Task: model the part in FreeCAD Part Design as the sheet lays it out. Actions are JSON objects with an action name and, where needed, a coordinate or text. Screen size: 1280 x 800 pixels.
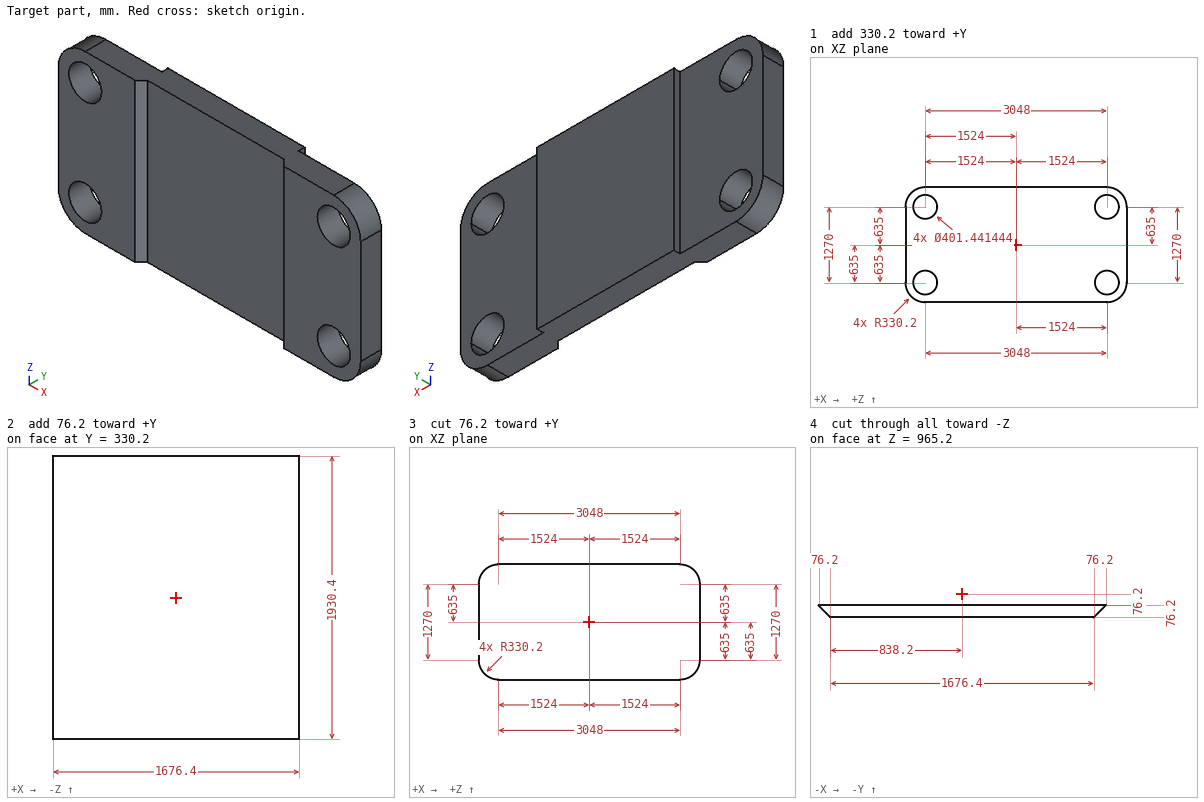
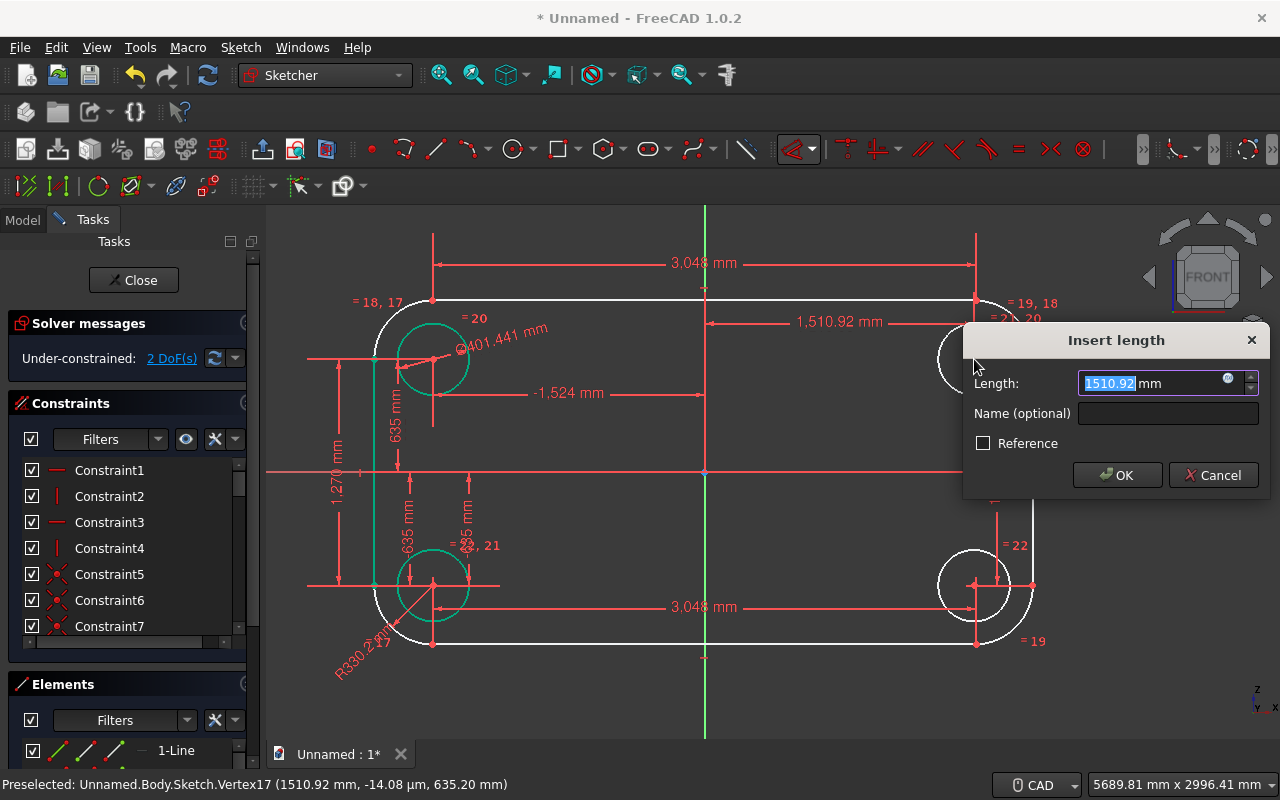
{"action": "type", "text": "1524"}
{"action": "key", "text": "Return"}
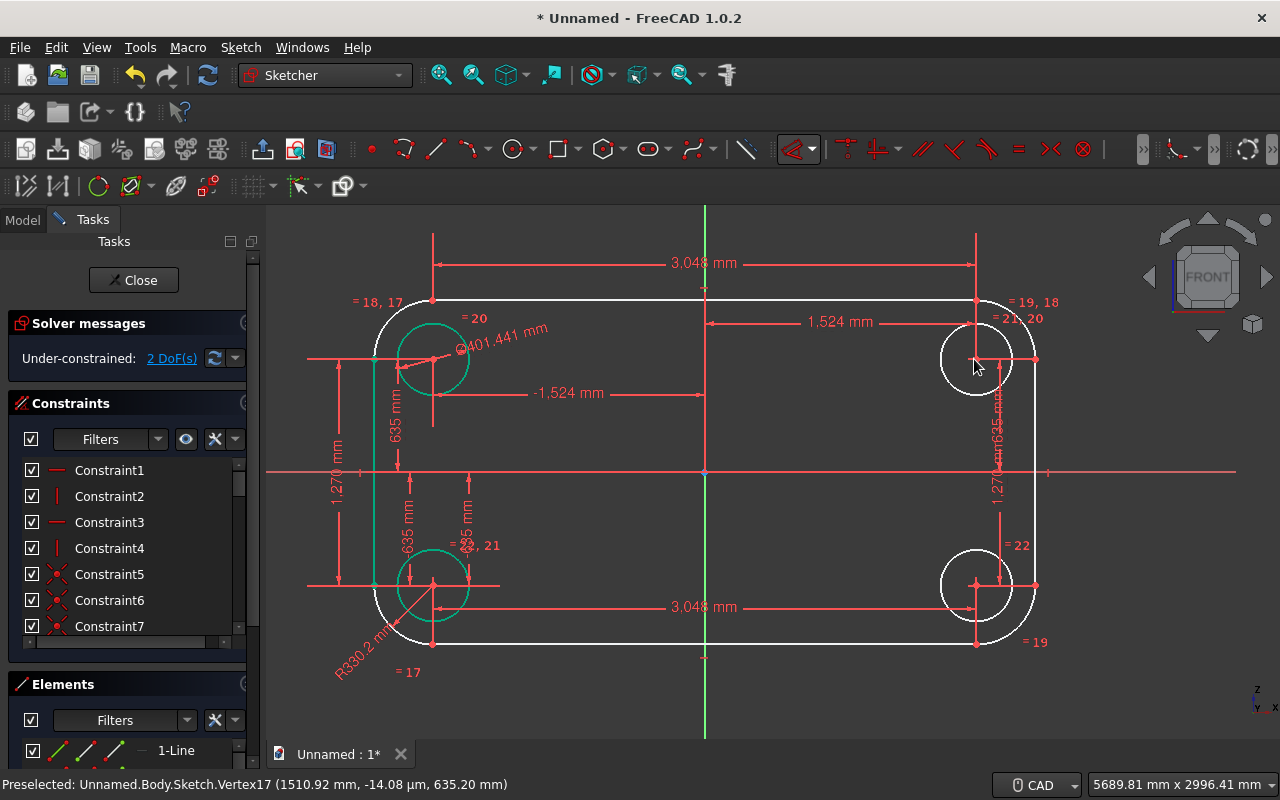
{"action": "left_click", "coordinate": [976, 644]}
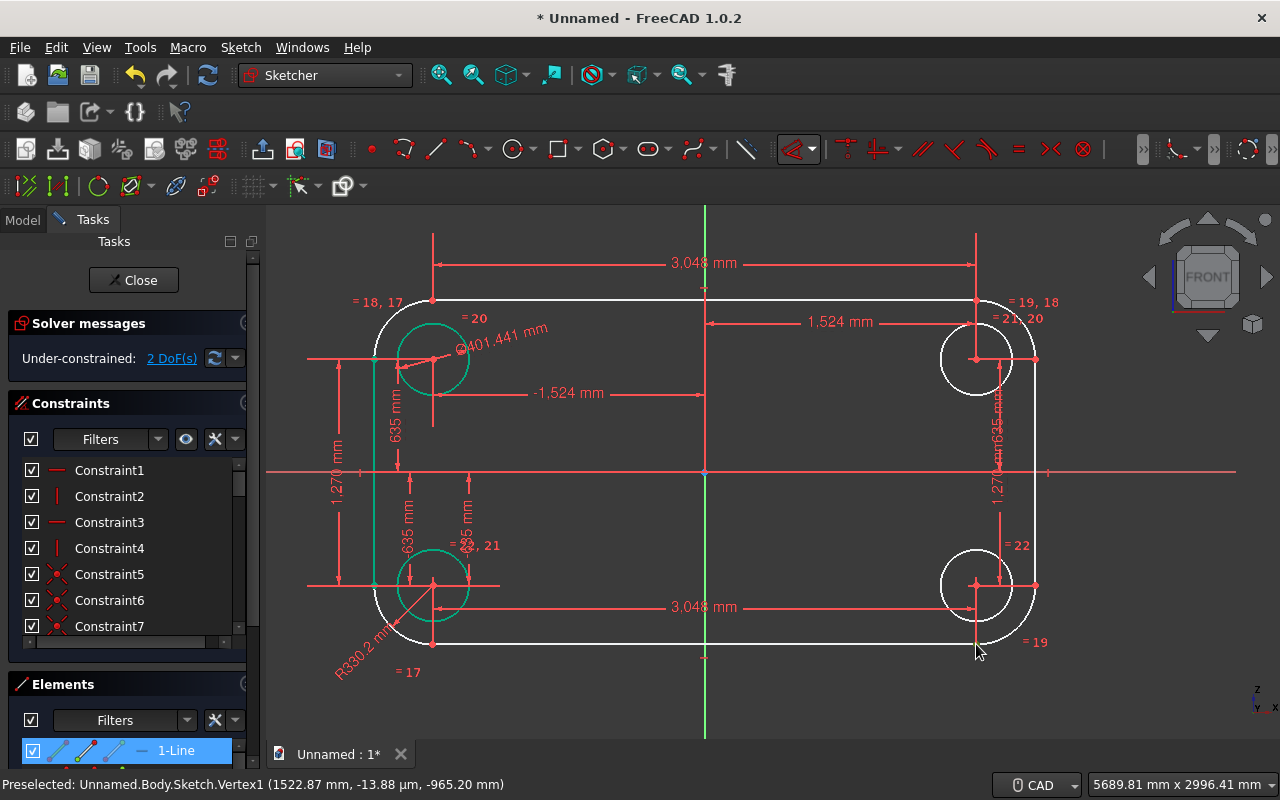
{"action": "key", "text": "l"}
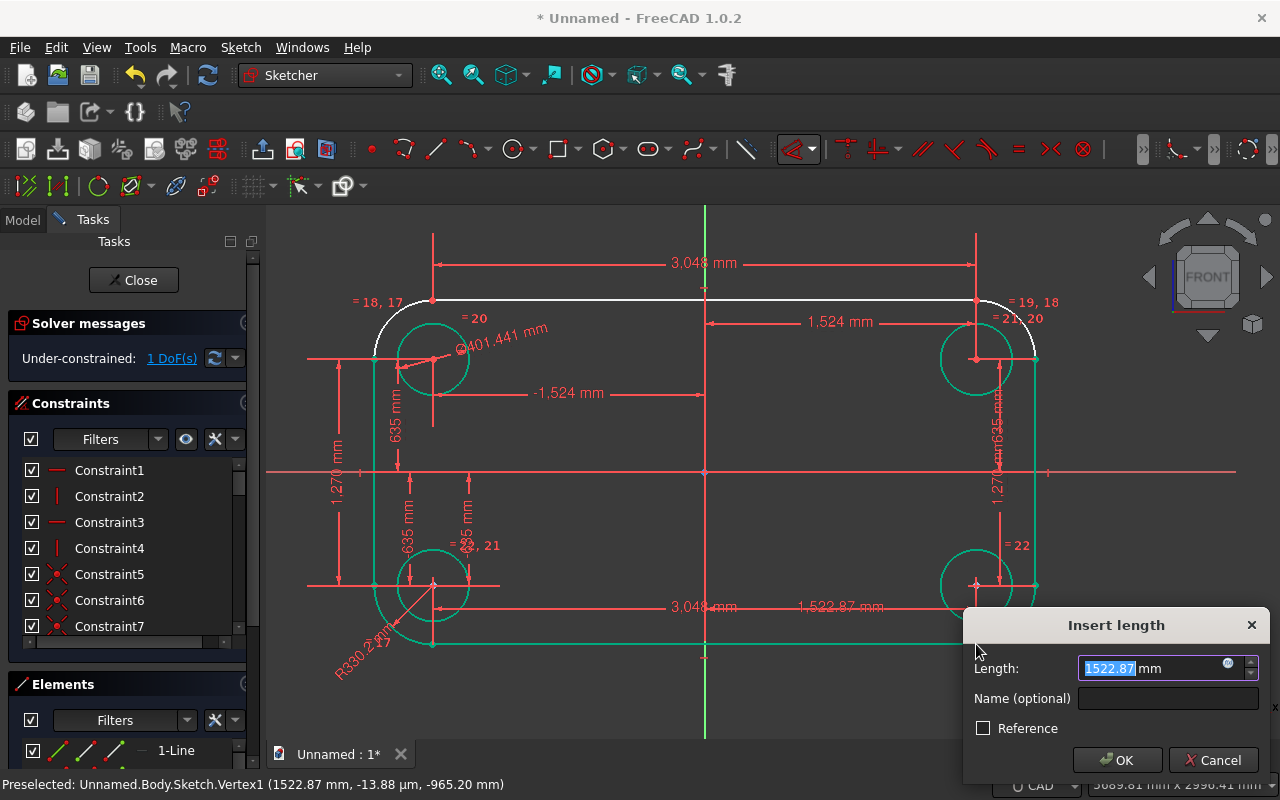
{"action": "type", "text": "1524"}
{"action": "key", "text": "Return"}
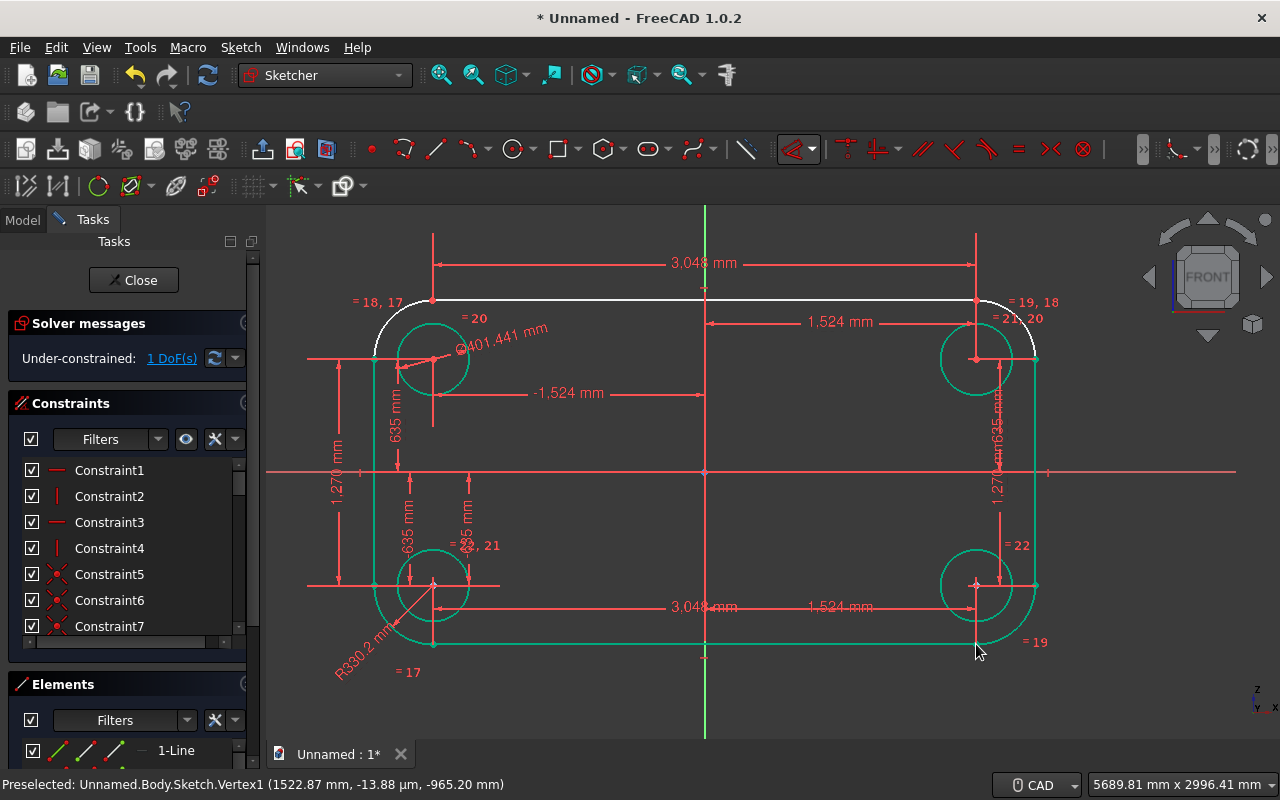
{"action": "left_click", "coordinate": [433, 300]}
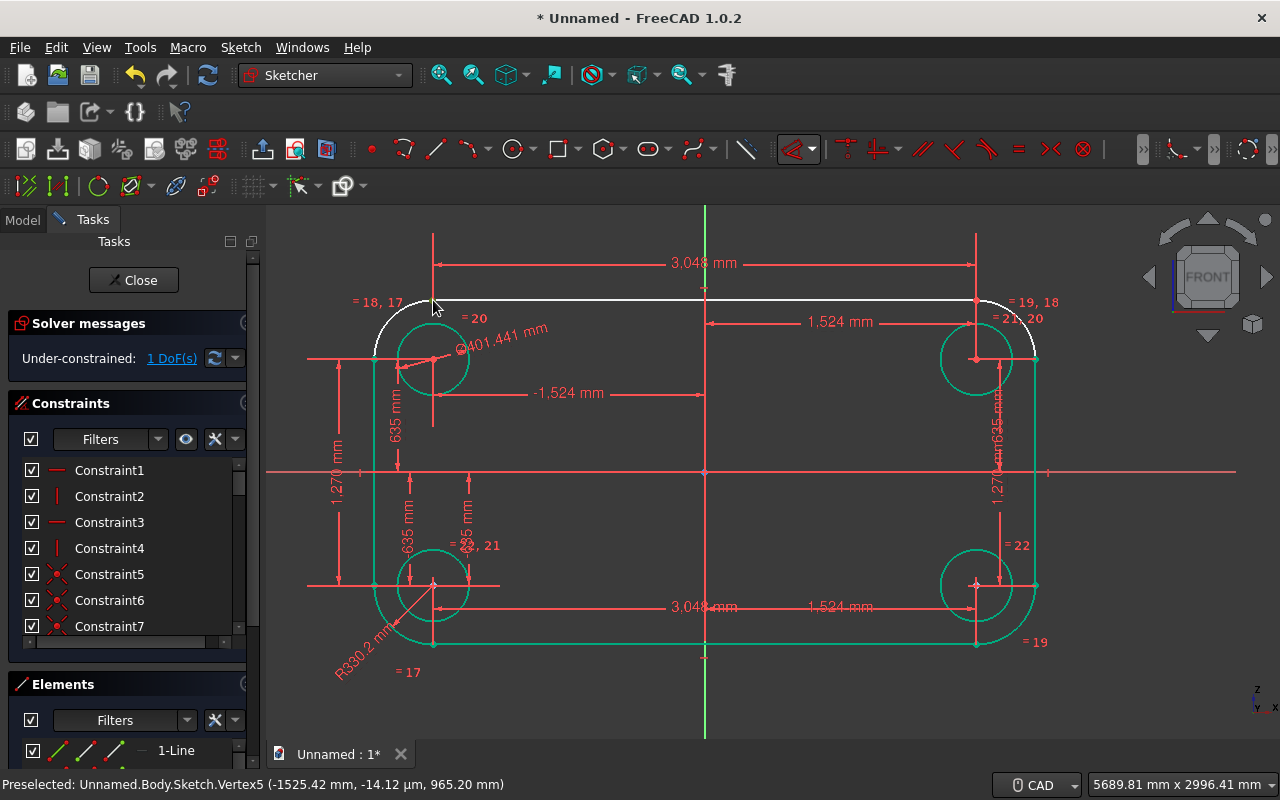
{"action": "left_click", "coordinate": [814, 150]}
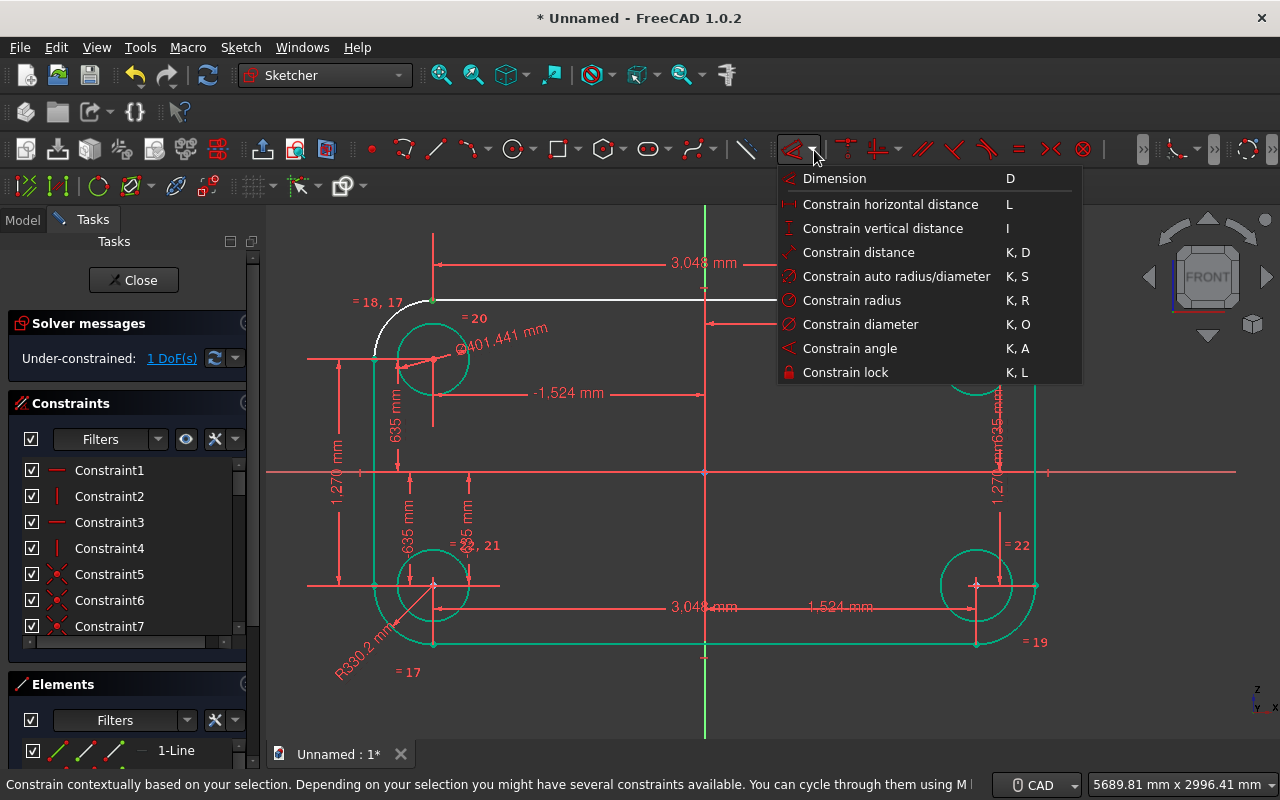
{"action": "left_click", "coordinate": [930, 204]}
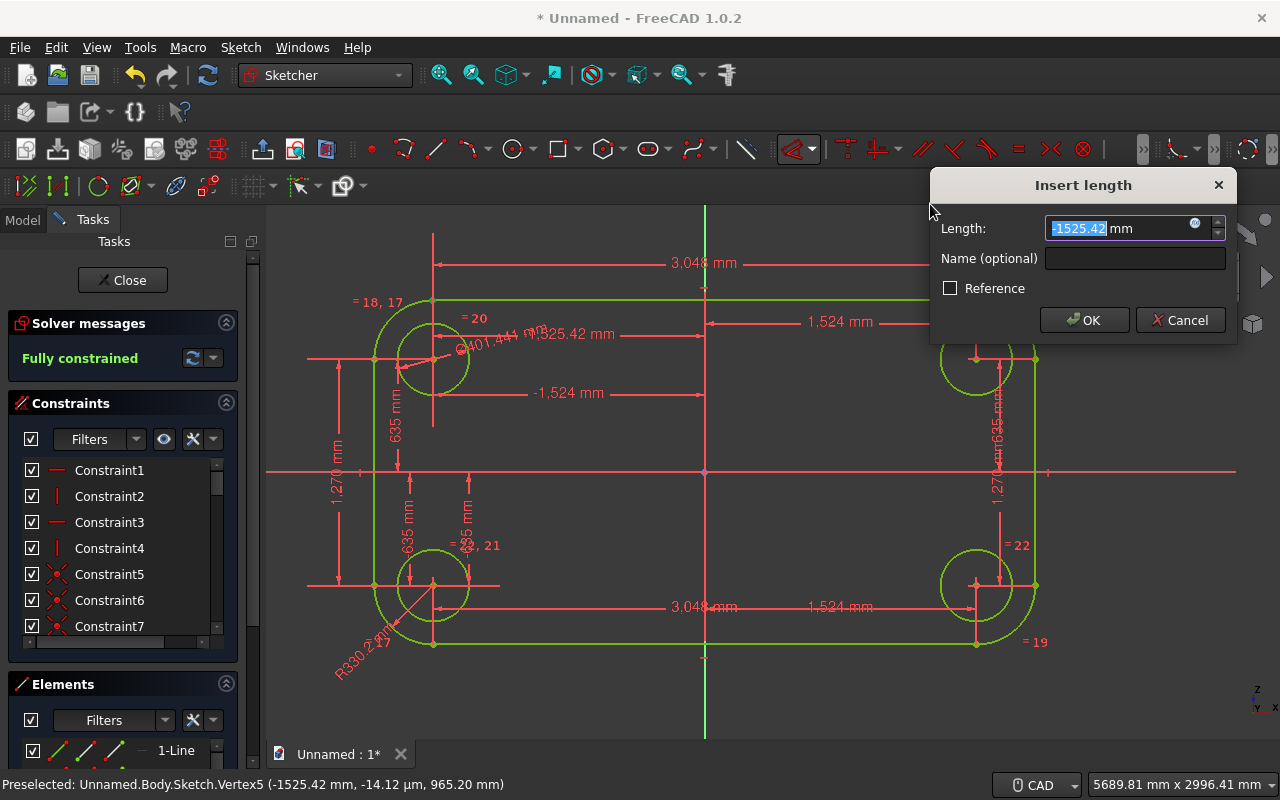
{"action": "type", "text": "-1524"}
{"action": "key", "text": "Return"}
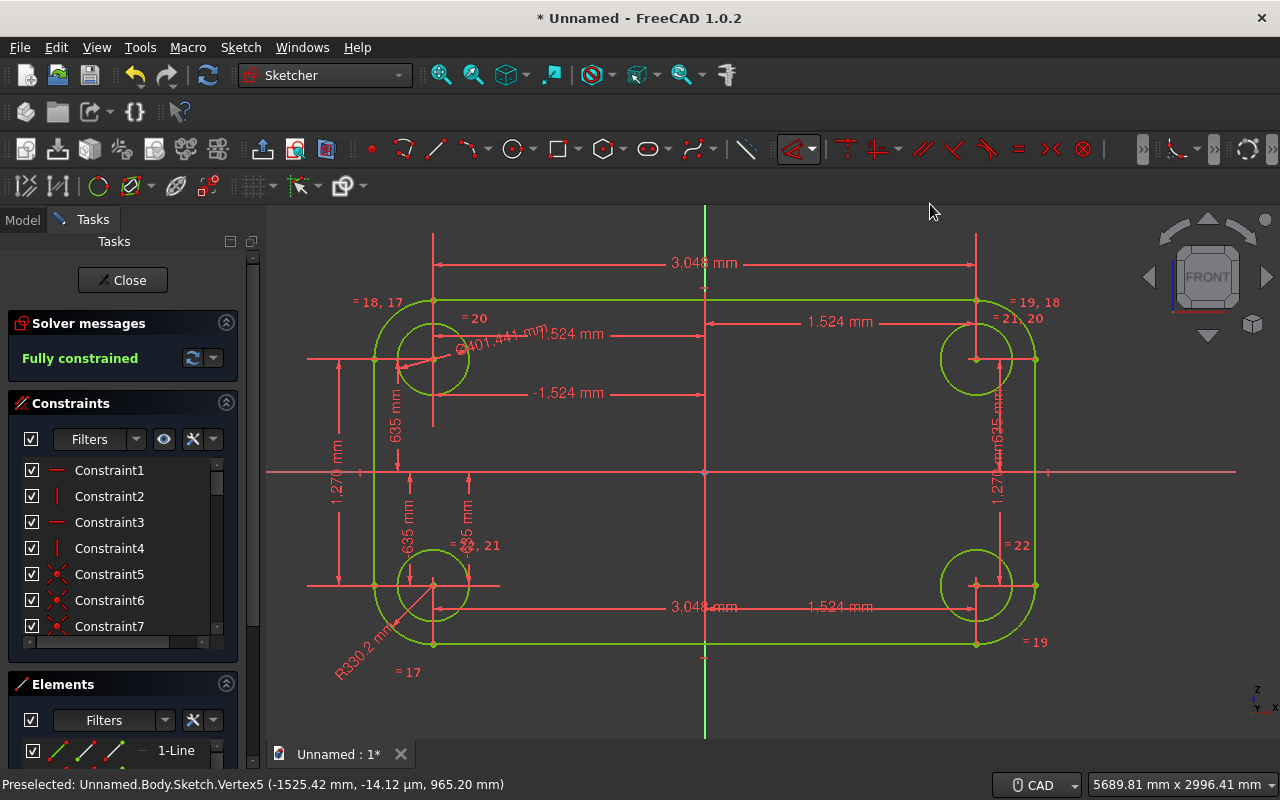
{"action": "left_click", "coordinate": [123, 280]}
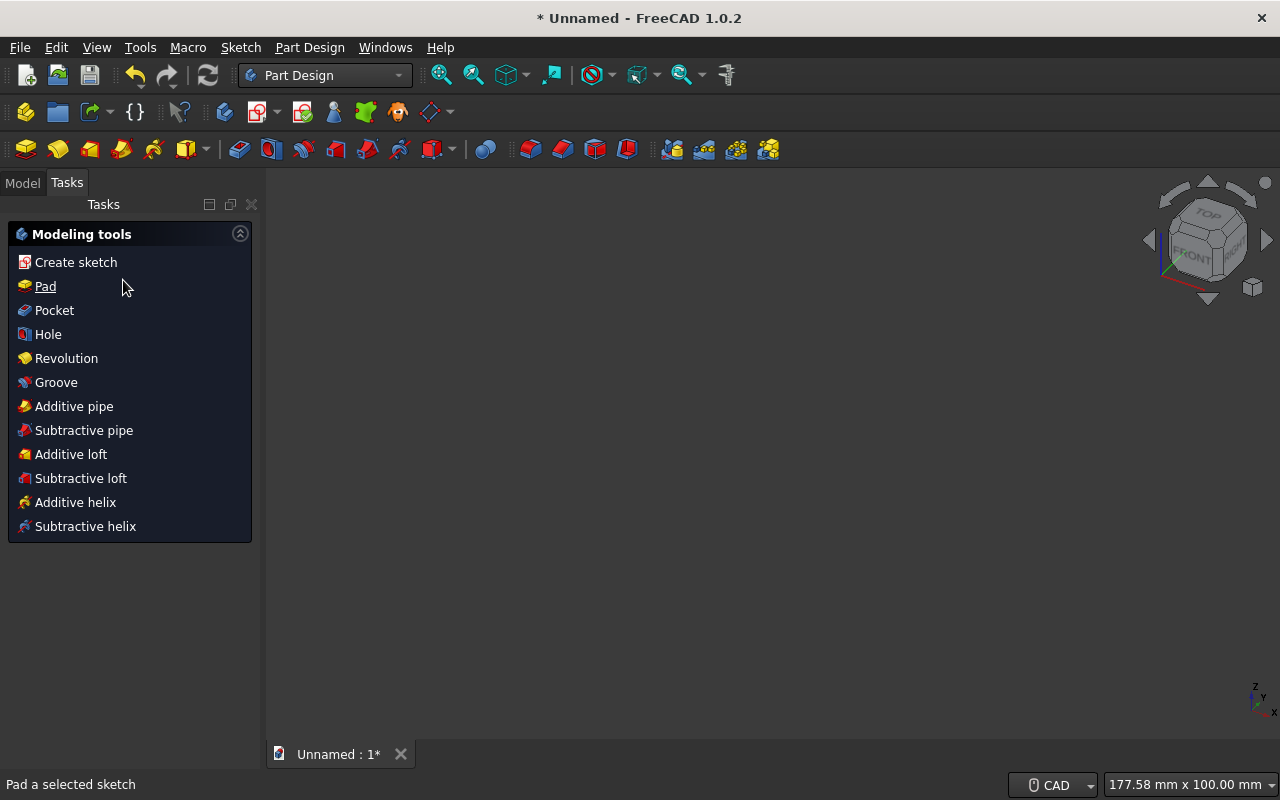
{"action": "left_click", "coordinate": [26, 150]}